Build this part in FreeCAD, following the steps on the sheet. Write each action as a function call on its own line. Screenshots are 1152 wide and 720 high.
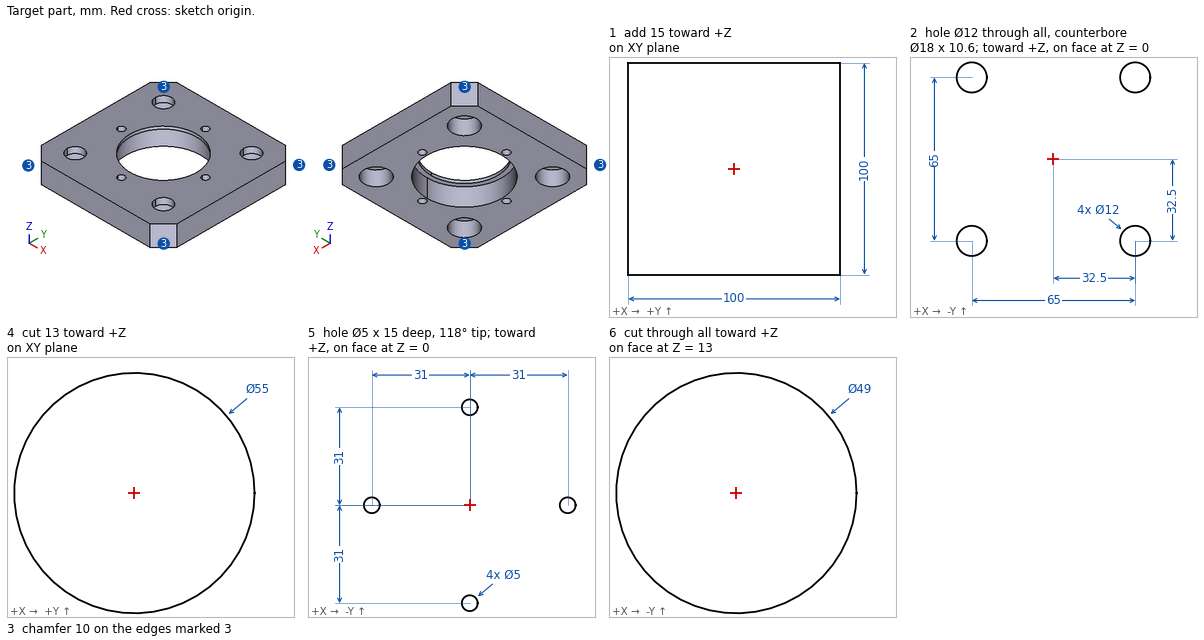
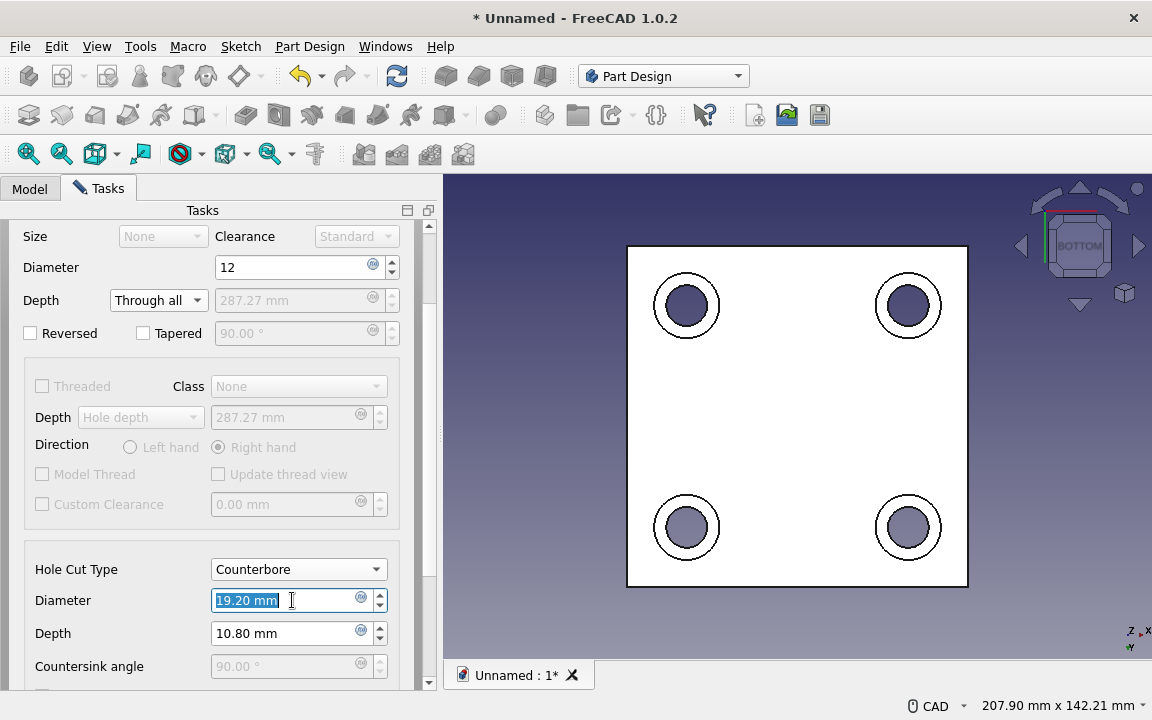
text(18)
key(Tab)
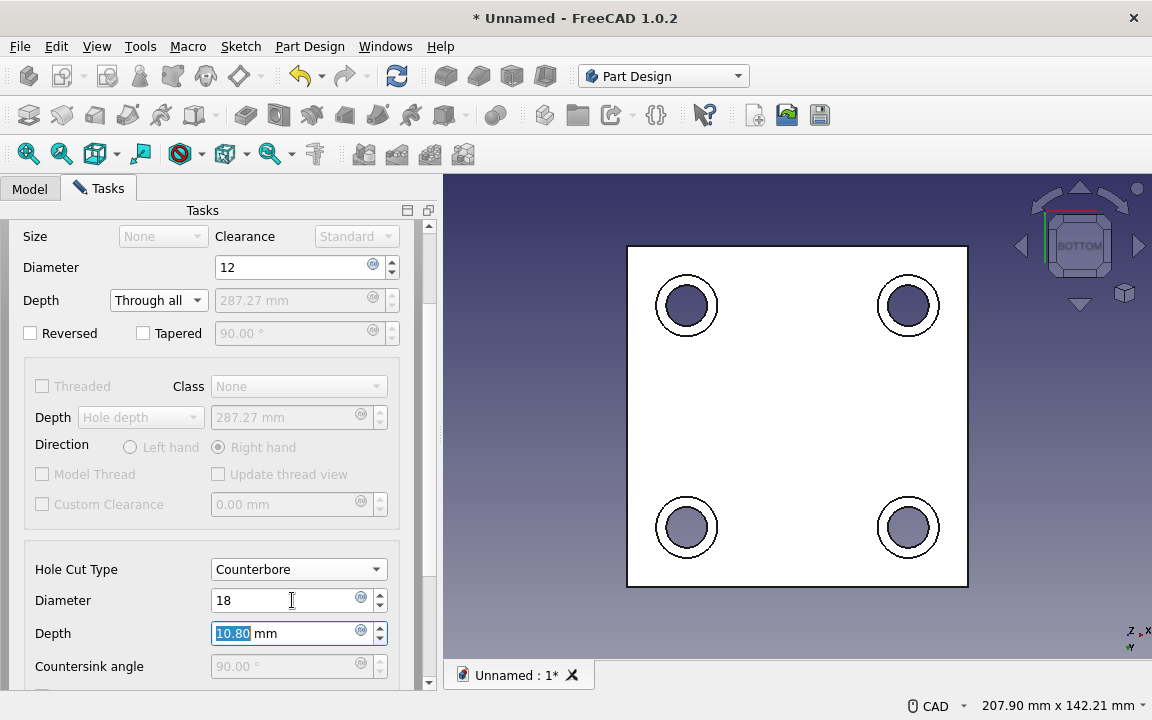
text(10.6)
key(Tab)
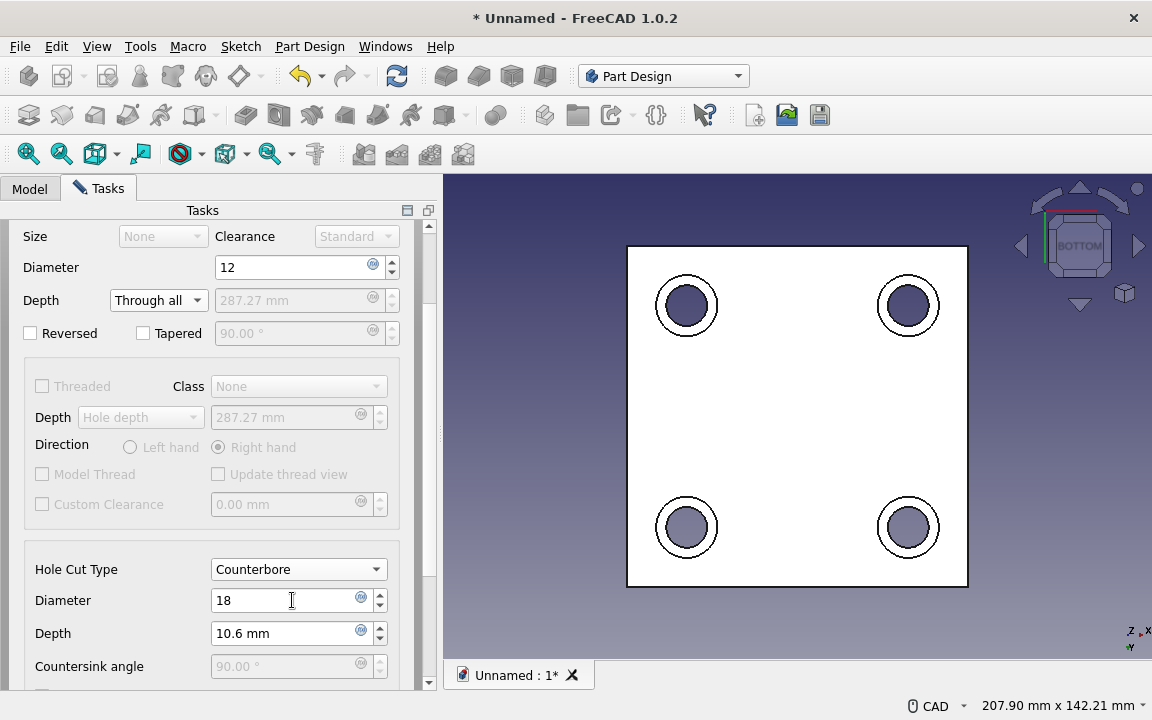
scroll(429, 455, up, 3)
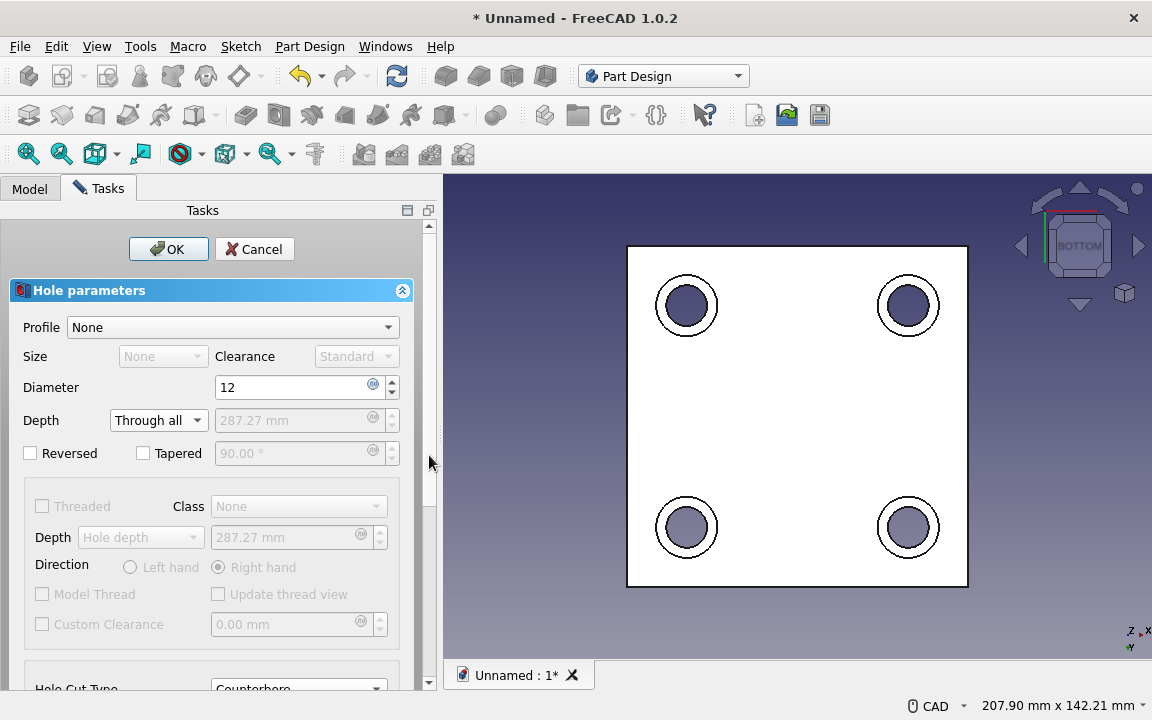
click(169, 249)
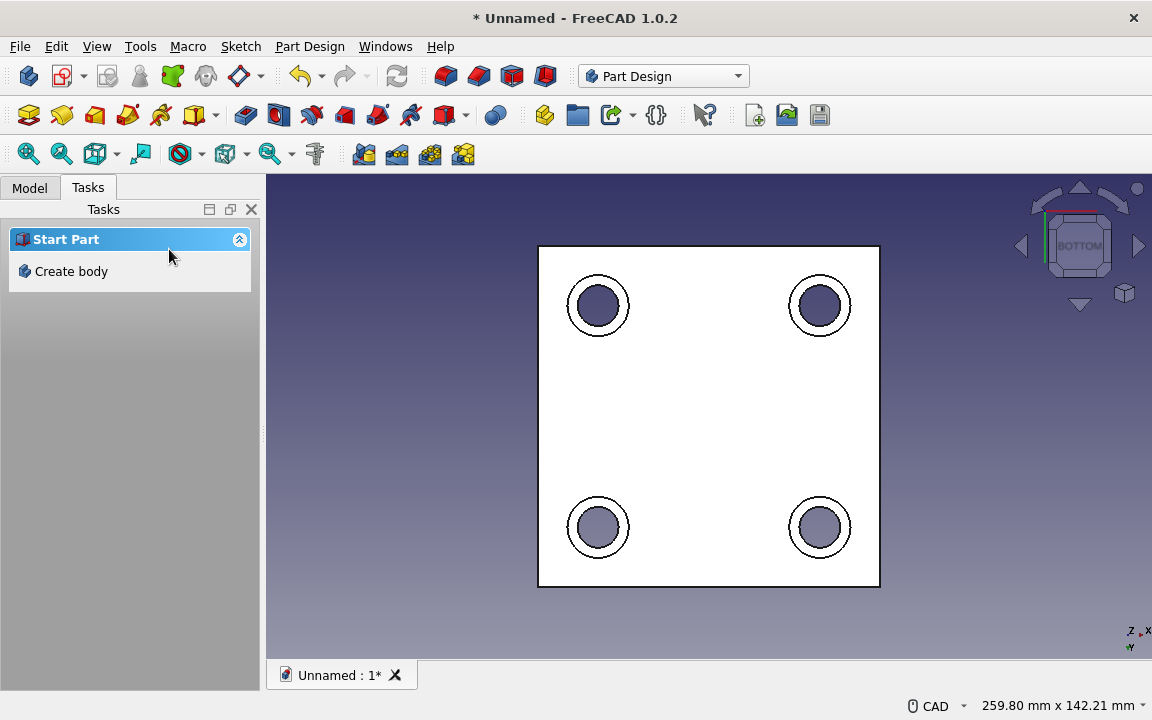
key(0)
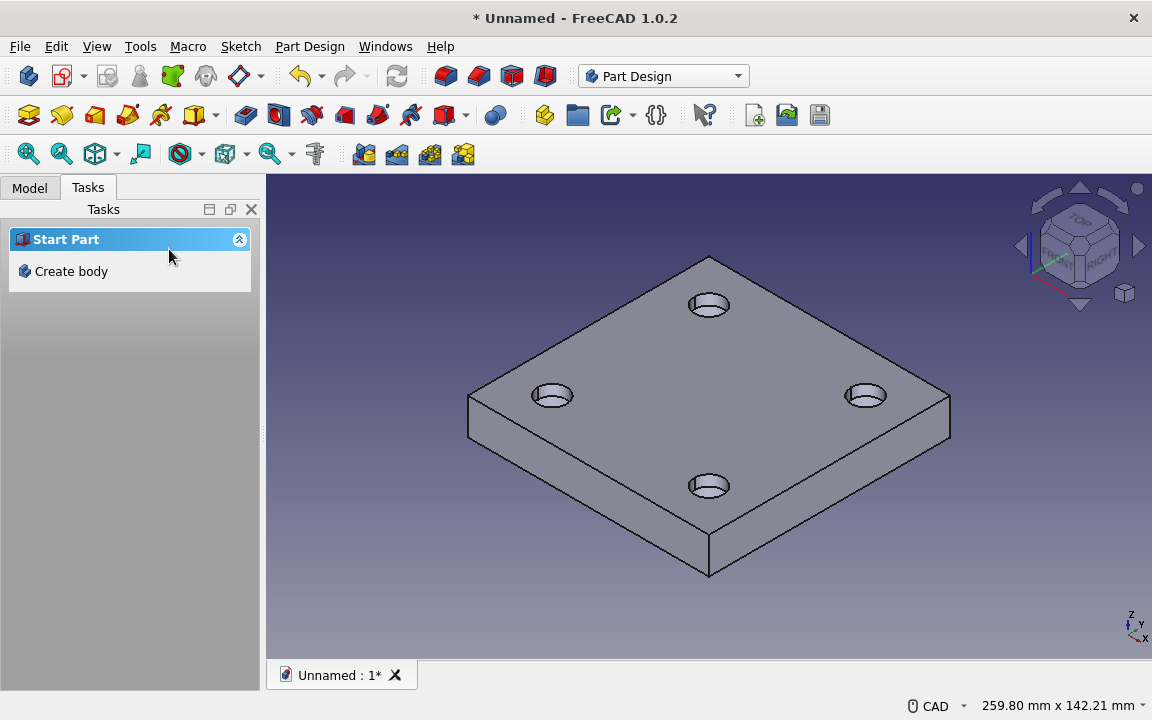
click(709, 555)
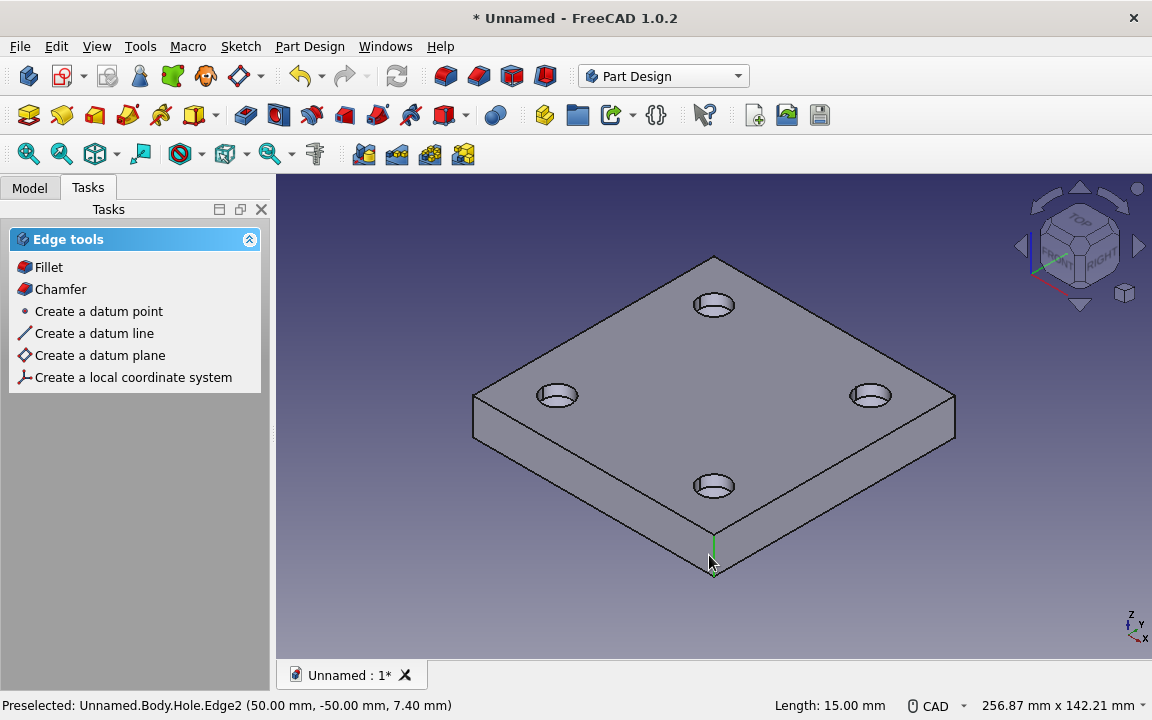
key(2)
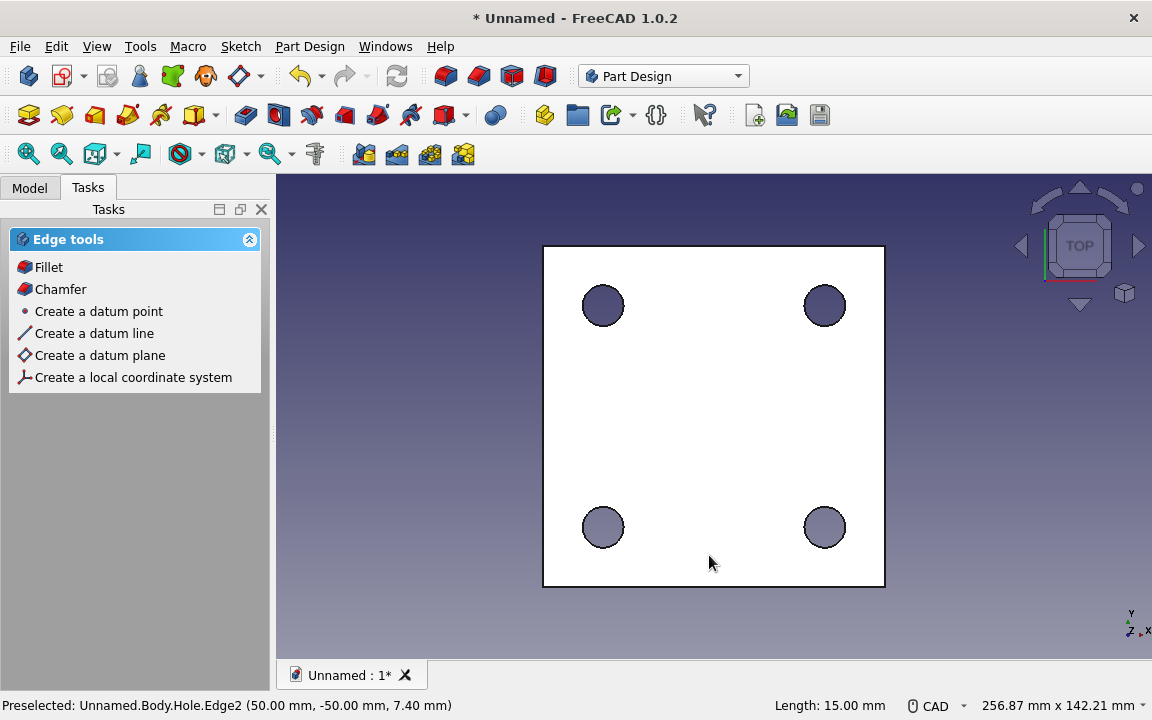
key(1)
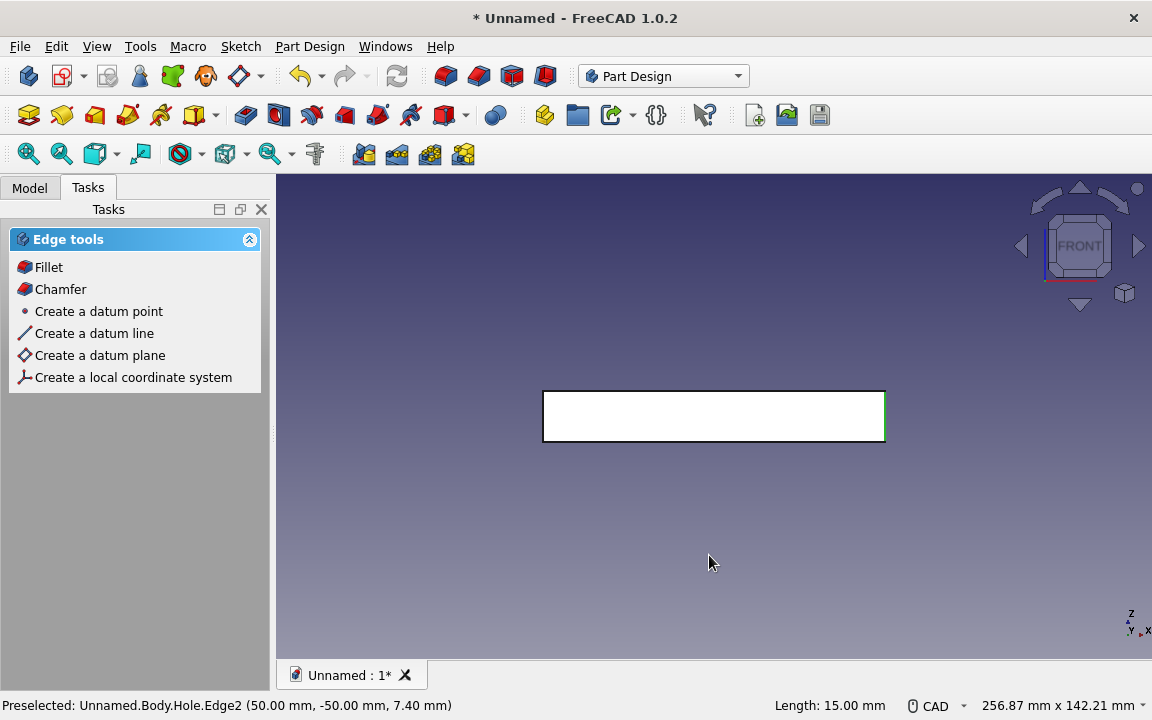
key(v)
key(f)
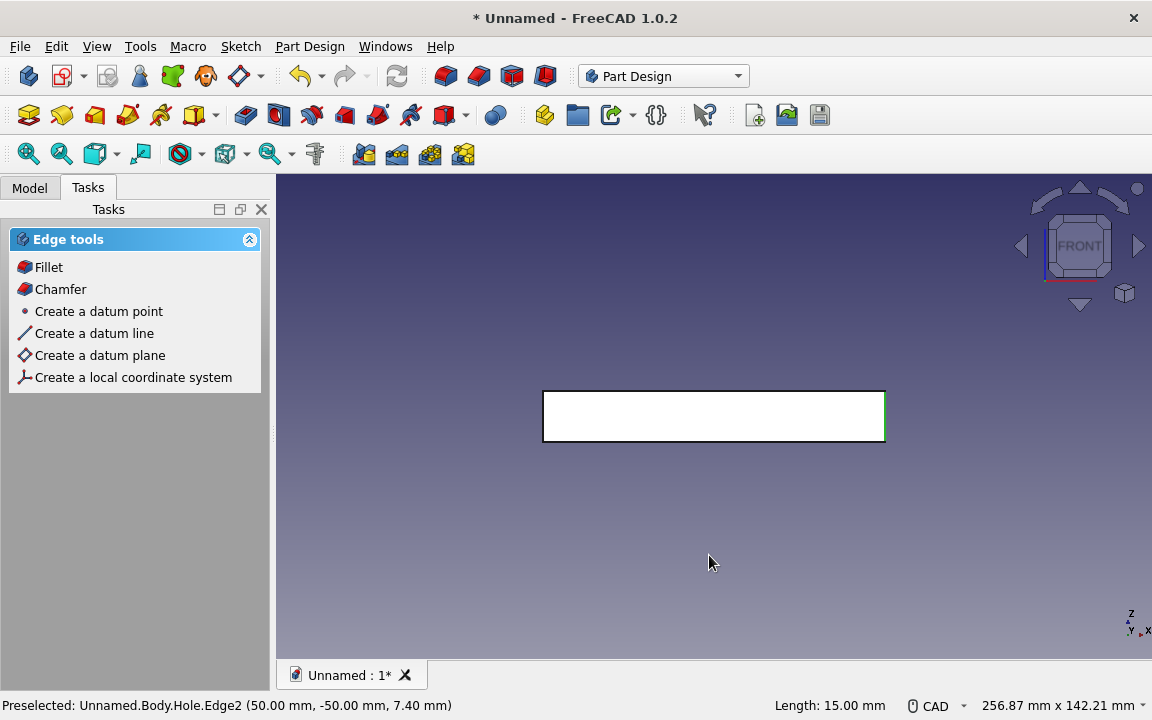
click(543, 416, ctrl)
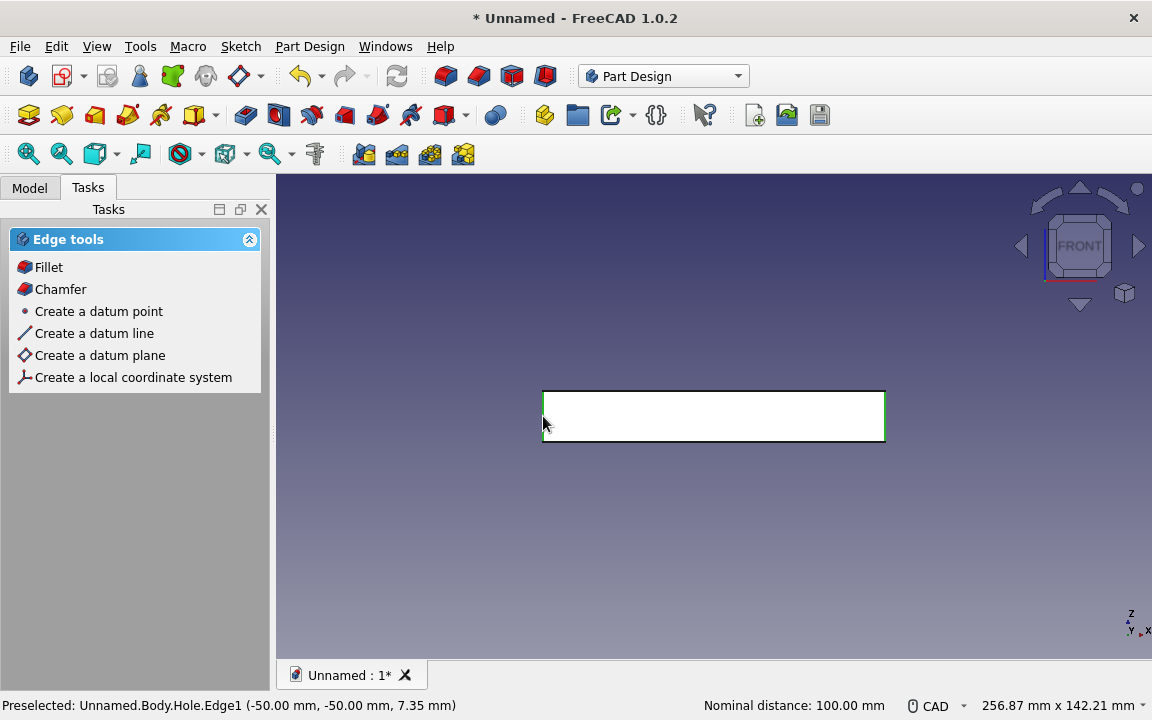
key(3)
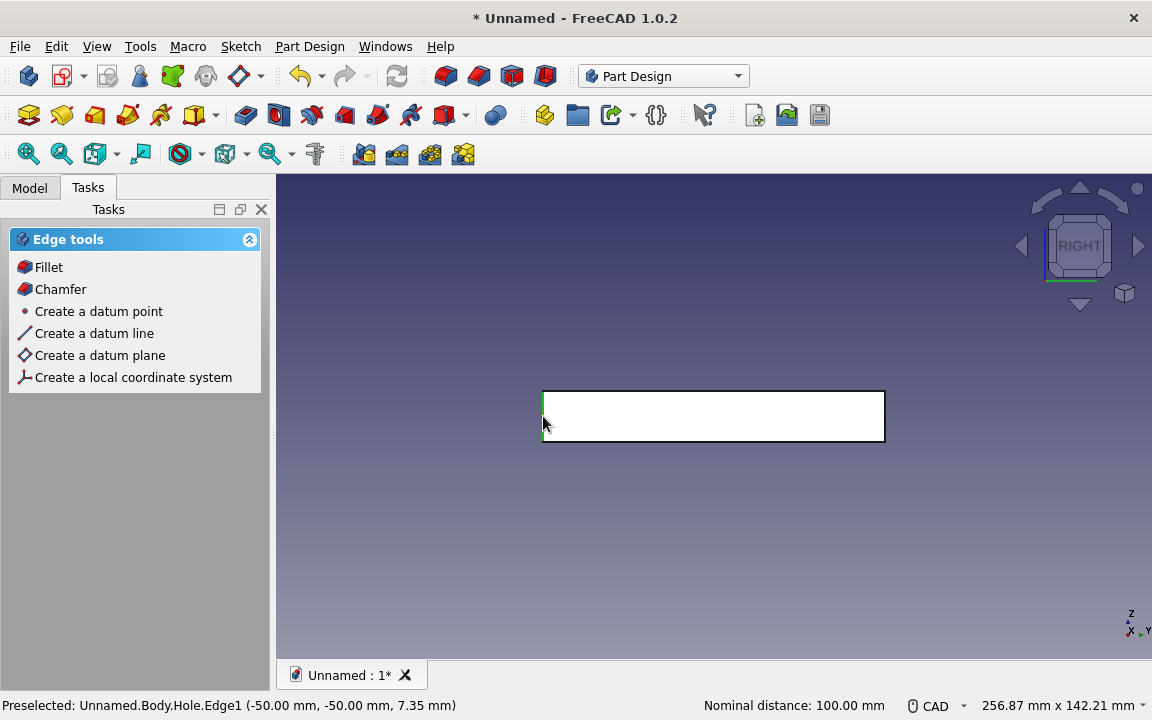
click(29, 154)